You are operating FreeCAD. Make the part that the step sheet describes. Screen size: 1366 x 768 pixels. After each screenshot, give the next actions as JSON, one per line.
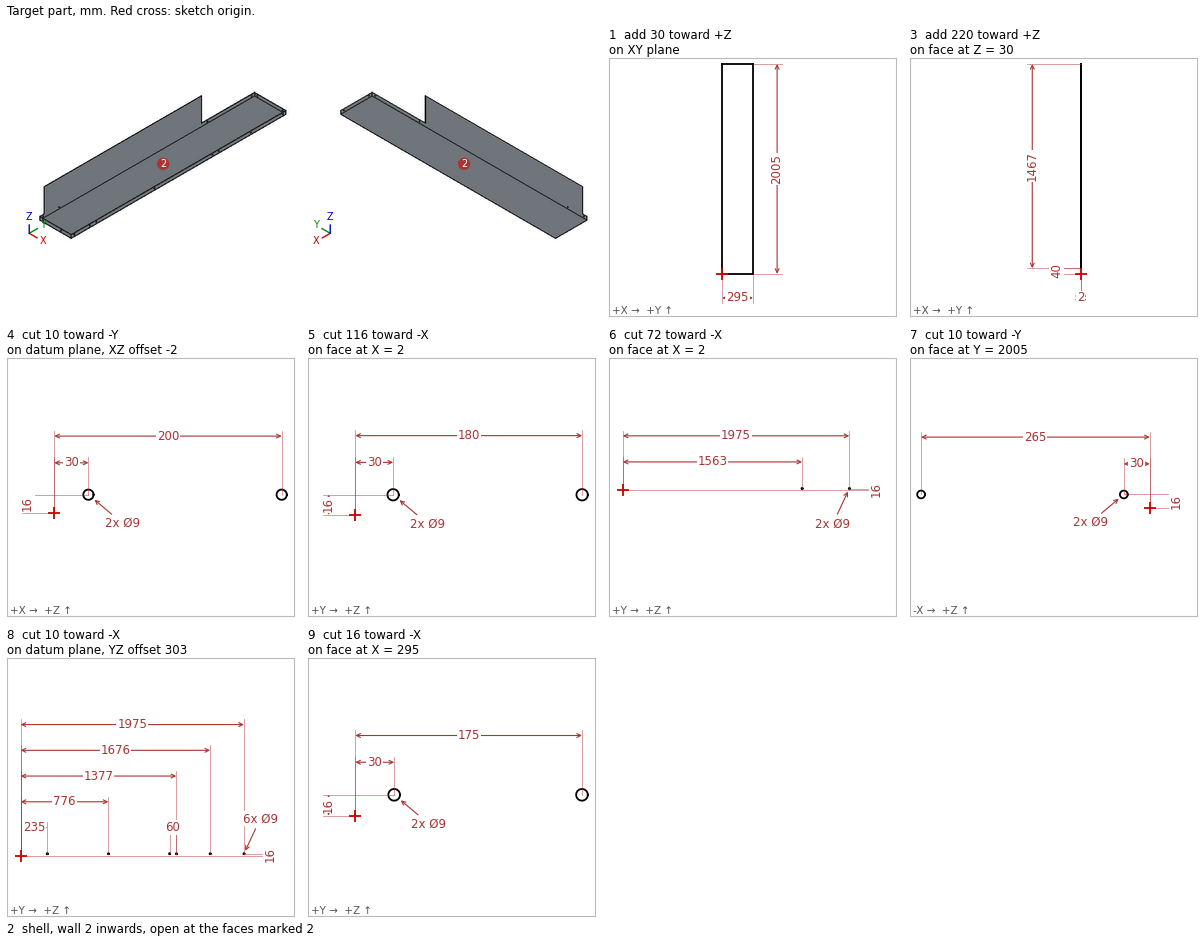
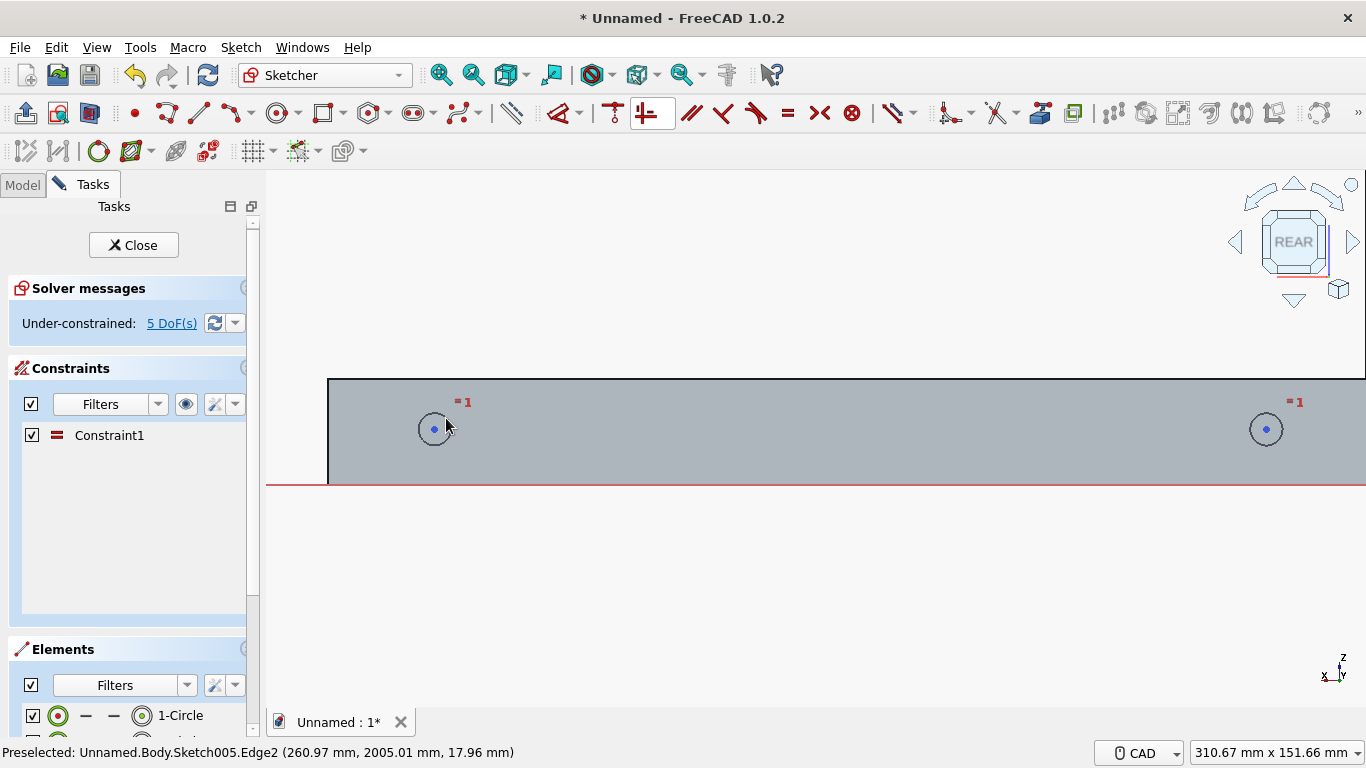
{"action": "scroll", "coordinate": [446, 418], "scroll_direction": "down", "scroll_amount": 2}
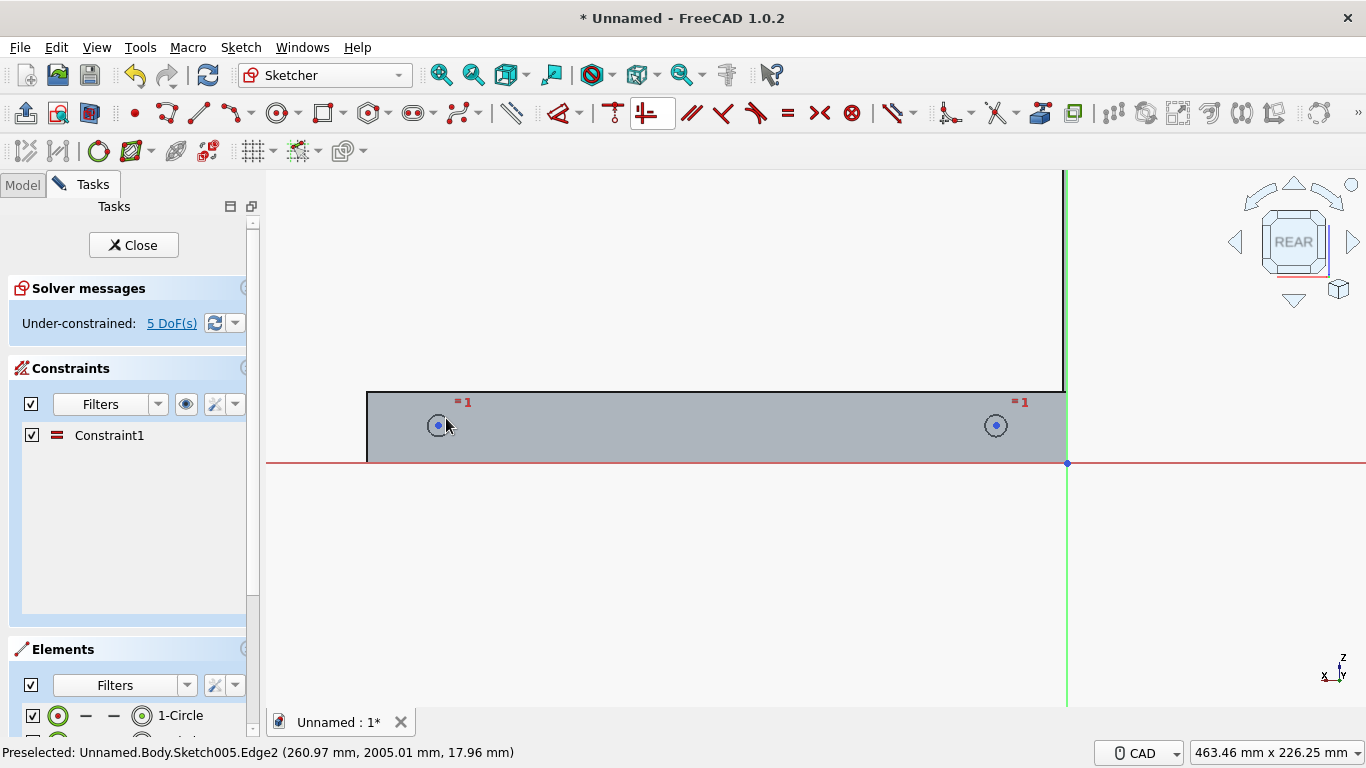
{"action": "left_click", "coordinate": [996, 426]}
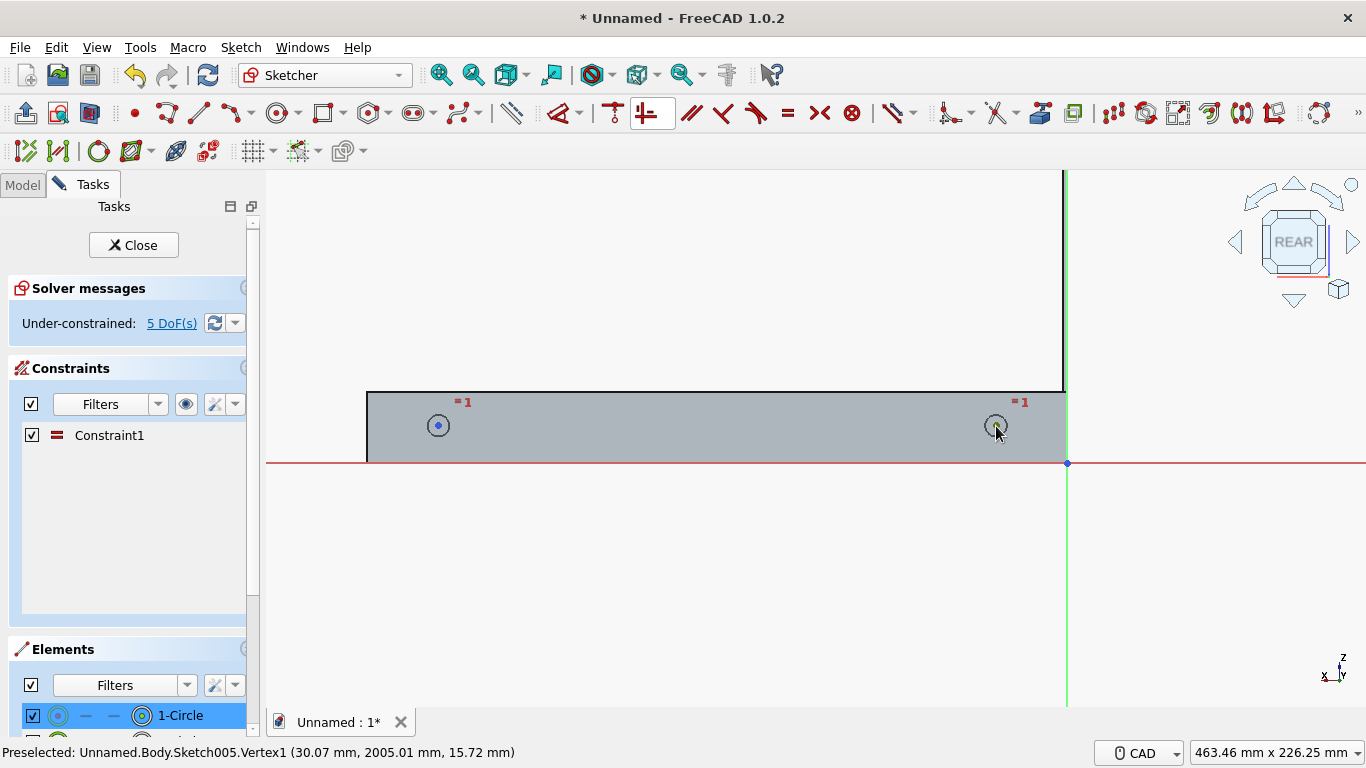
{"action": "left_click", "coordinate": [439, 426]}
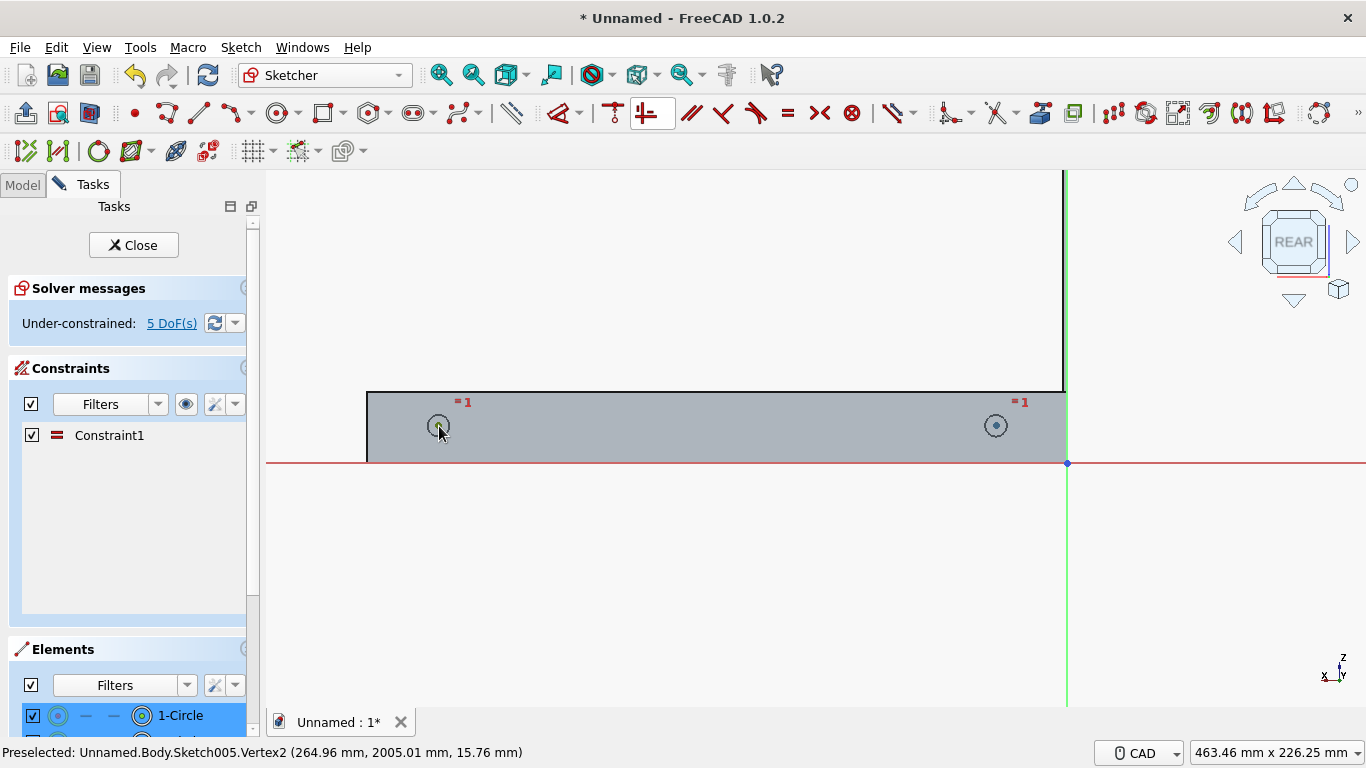
{"action": "left_click", "coordinate": [670, 114]}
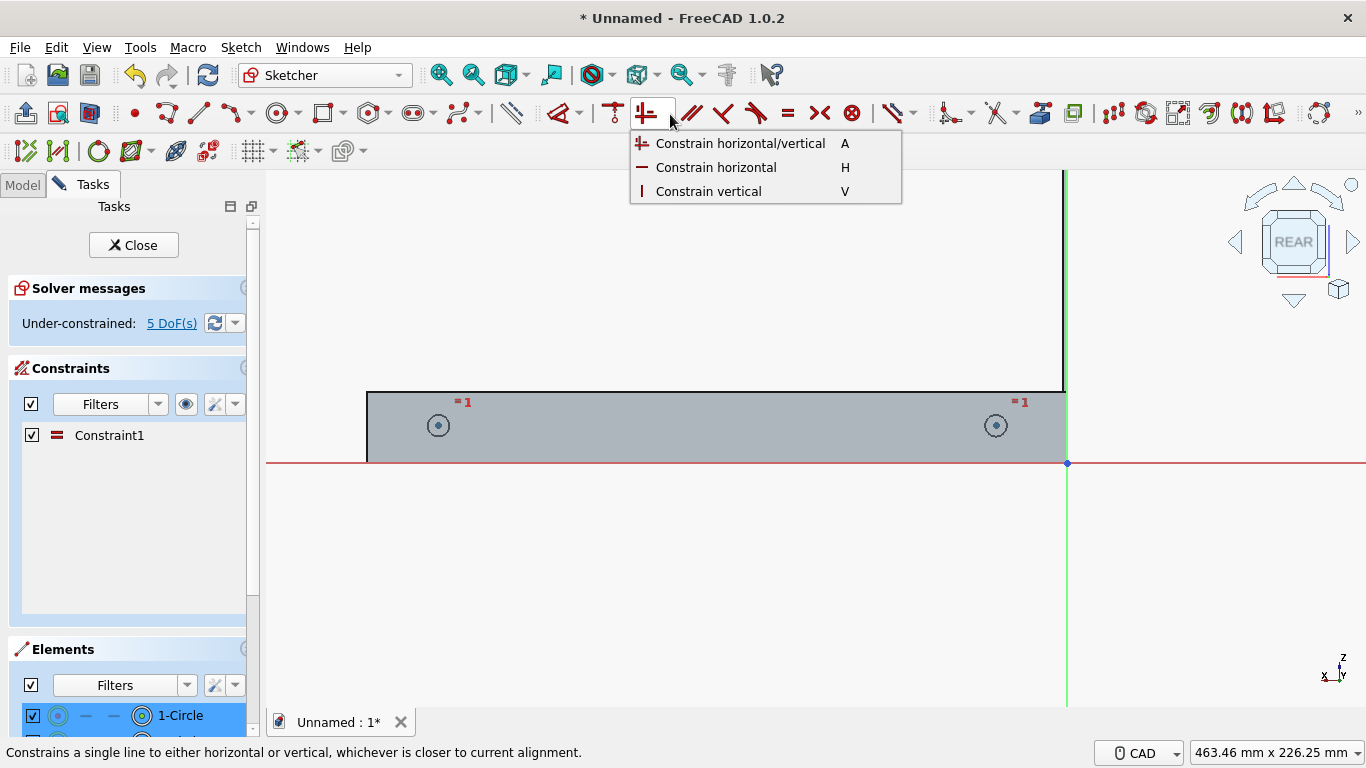
{"action": "left_click", "coordinate": [766, 167]}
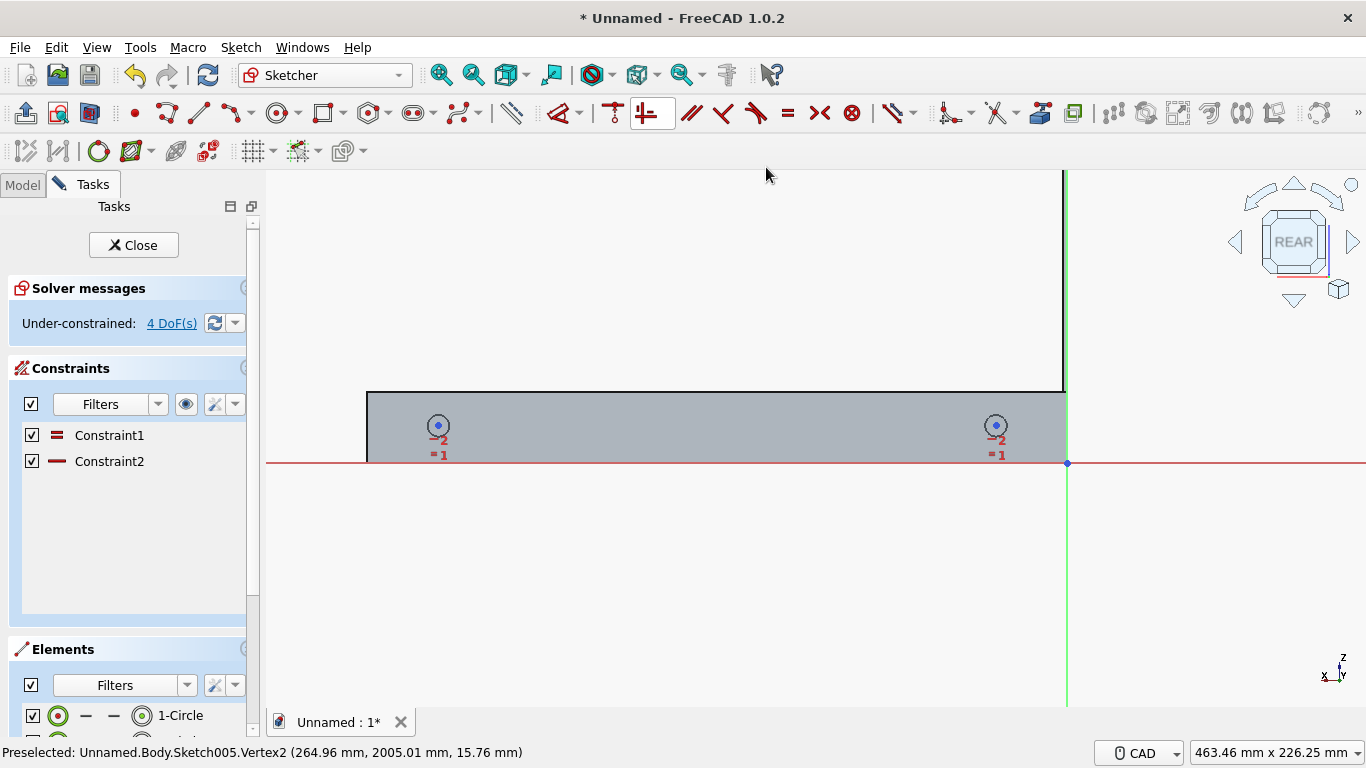
{"action": "left_click", "coordinate": [558, 114]}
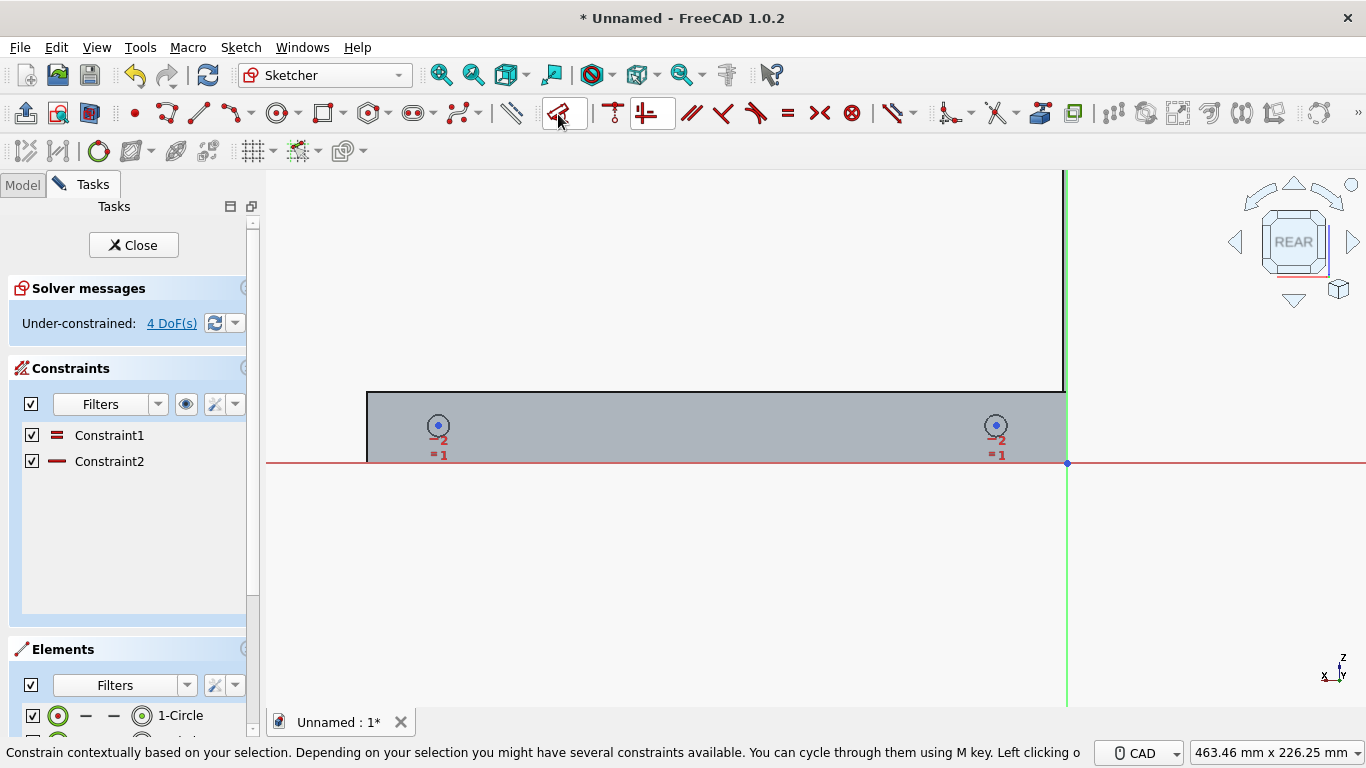
{"action": "scroll", "coordinate": [1004, 418], "scroll_direction": "up", "scroll_amount": 4}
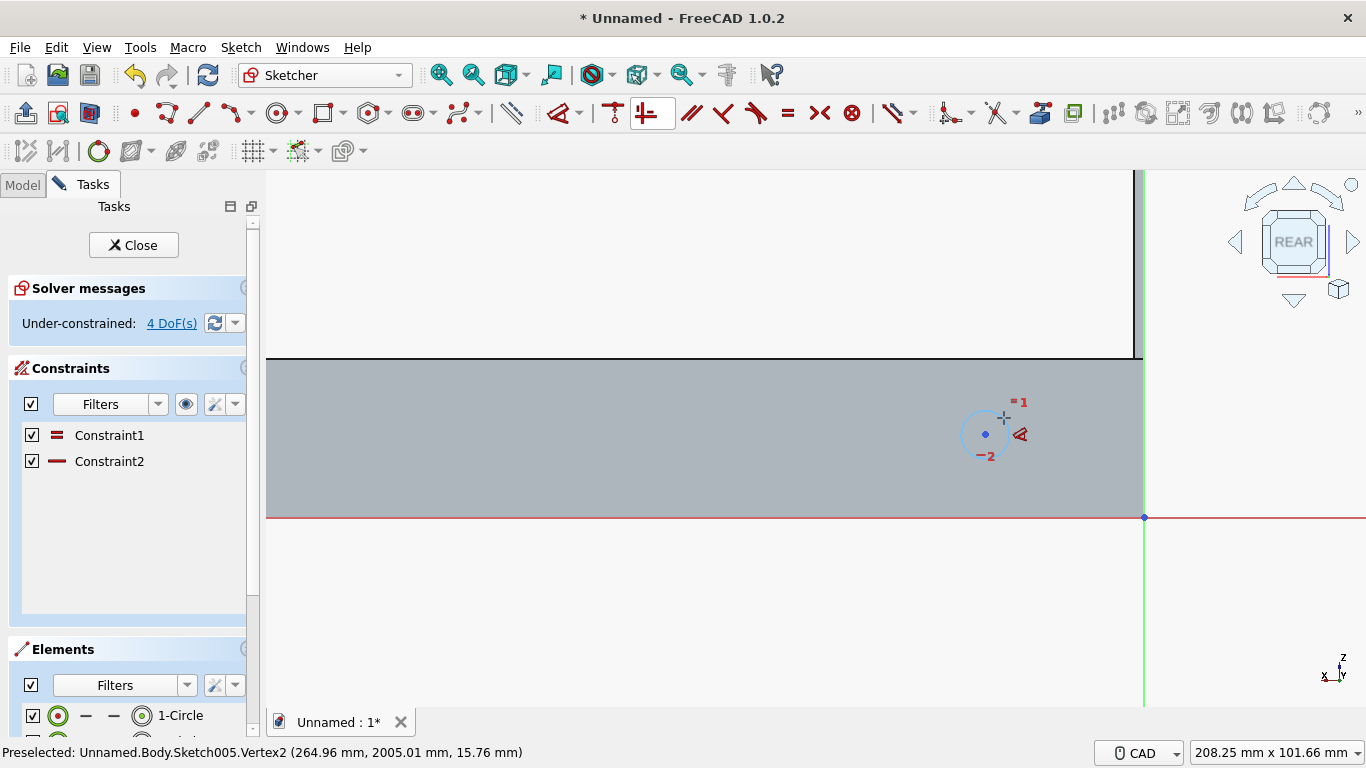
{"action": "left_click", "coordinate": [1002, 418]}
{"action": "left_click", "coordinate": [1024, 395]}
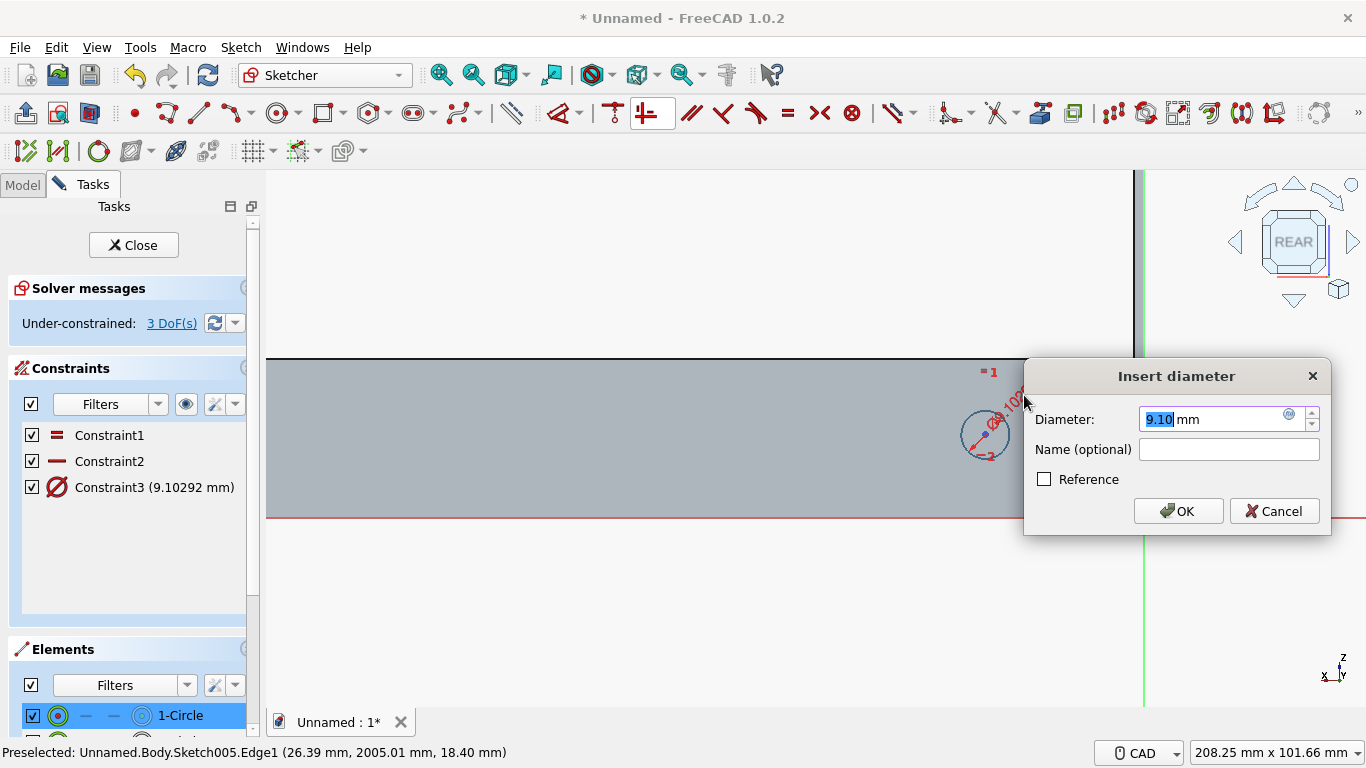
{"action": "type", "text": "9"}
{"action": "key", "text": "Return"}